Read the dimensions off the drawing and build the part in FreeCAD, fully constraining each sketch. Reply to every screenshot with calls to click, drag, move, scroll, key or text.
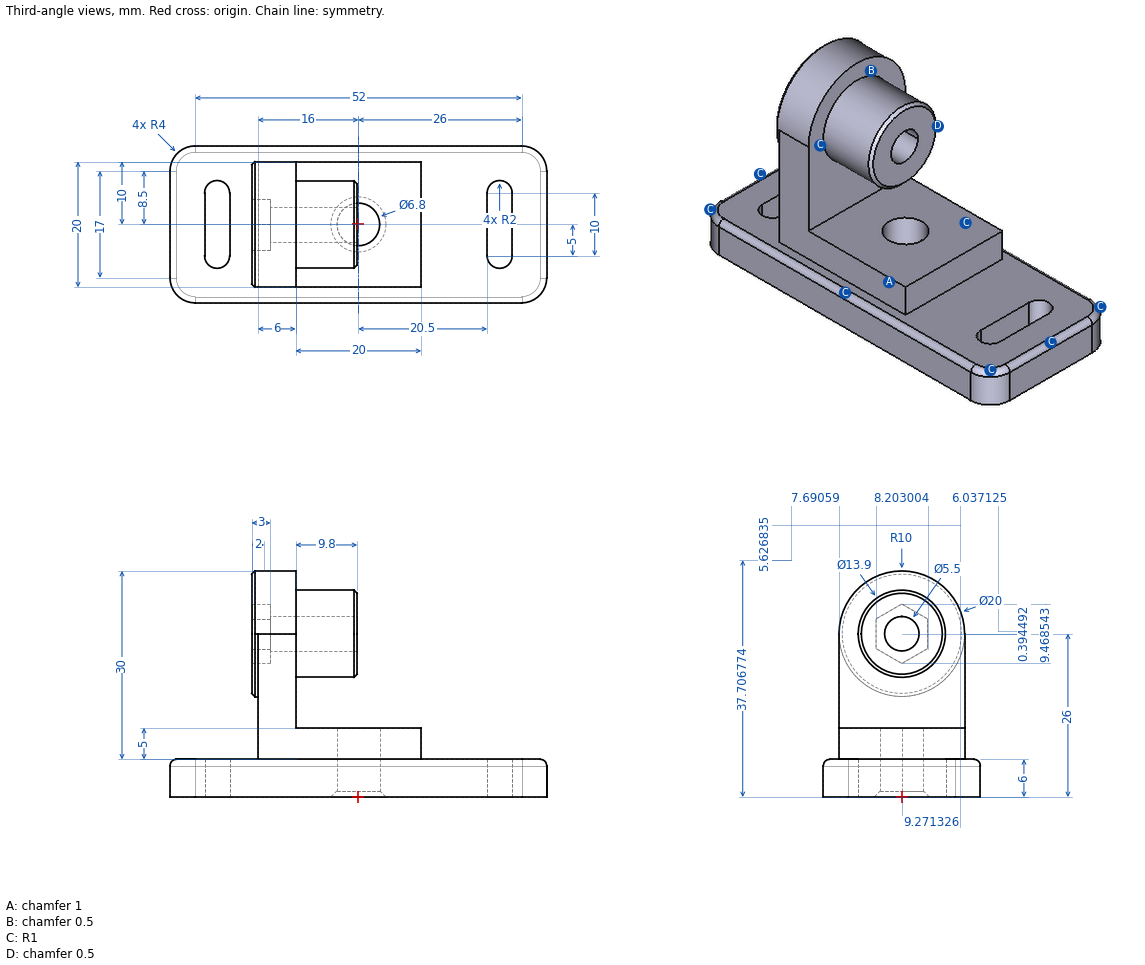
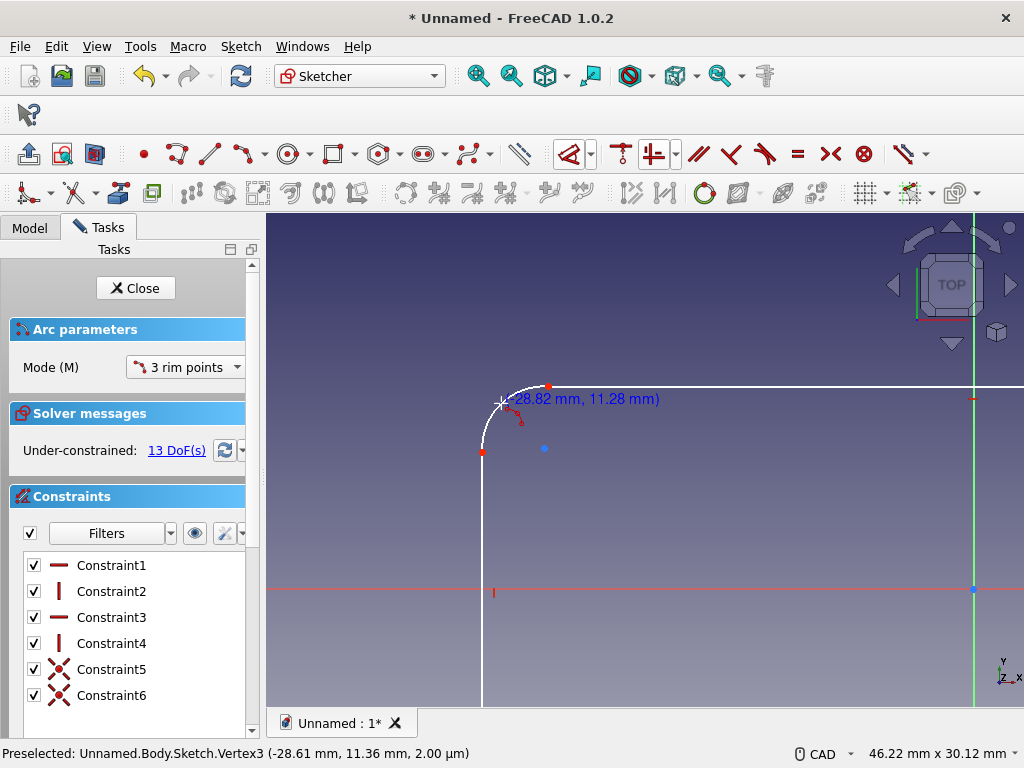
scroll(345, 385, down, 5)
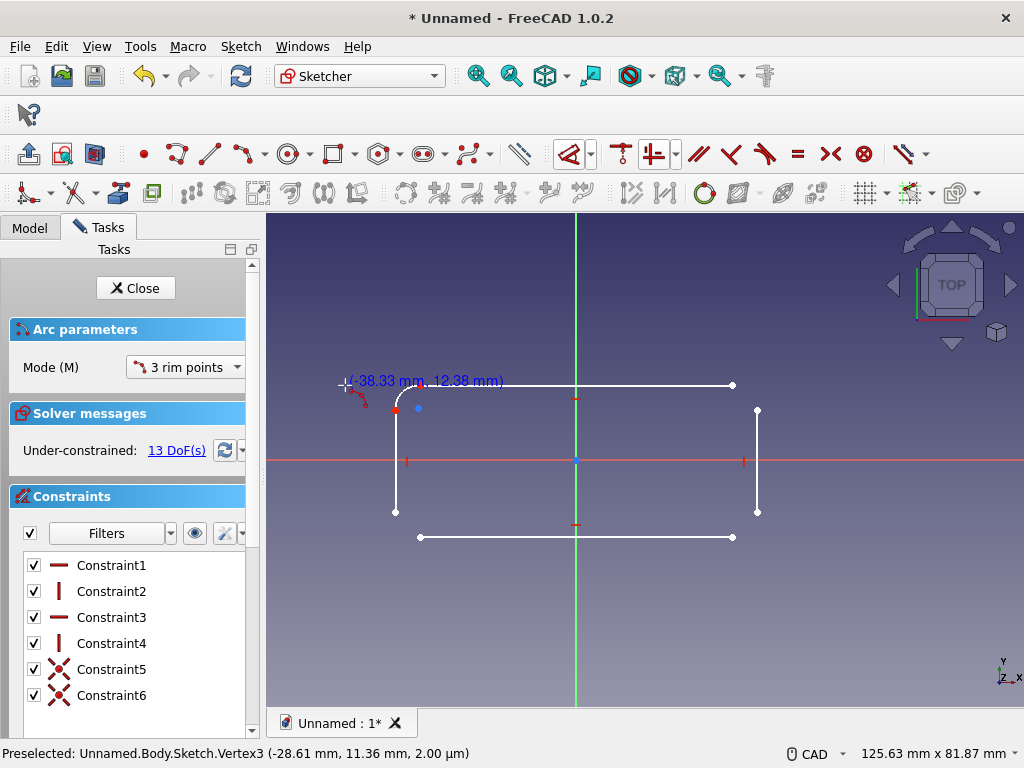
click(396, 513)
click(420, 537)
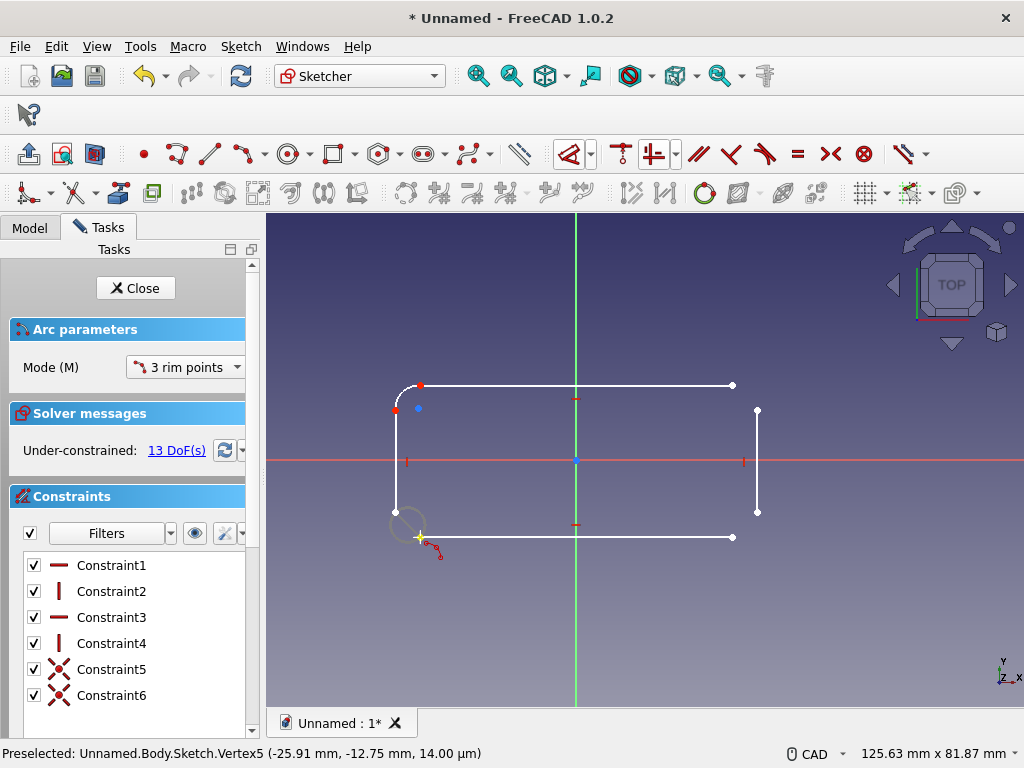
scroll(402, 529, up, 5)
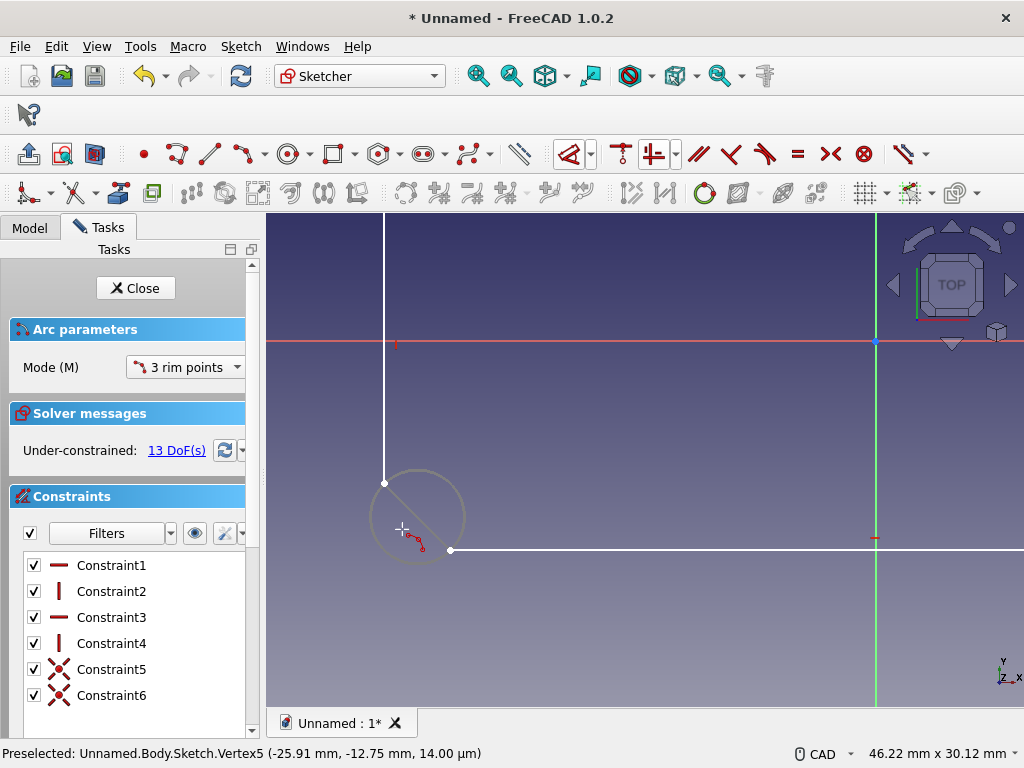
click(403, 527)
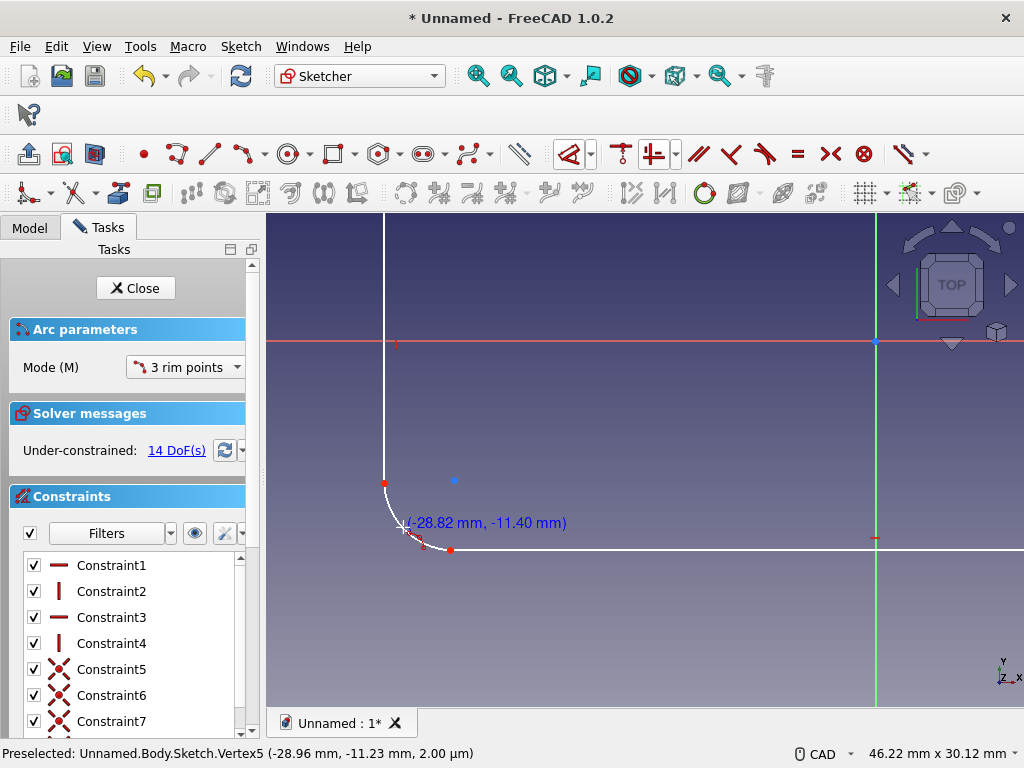
scroll(402, 529, down, 5)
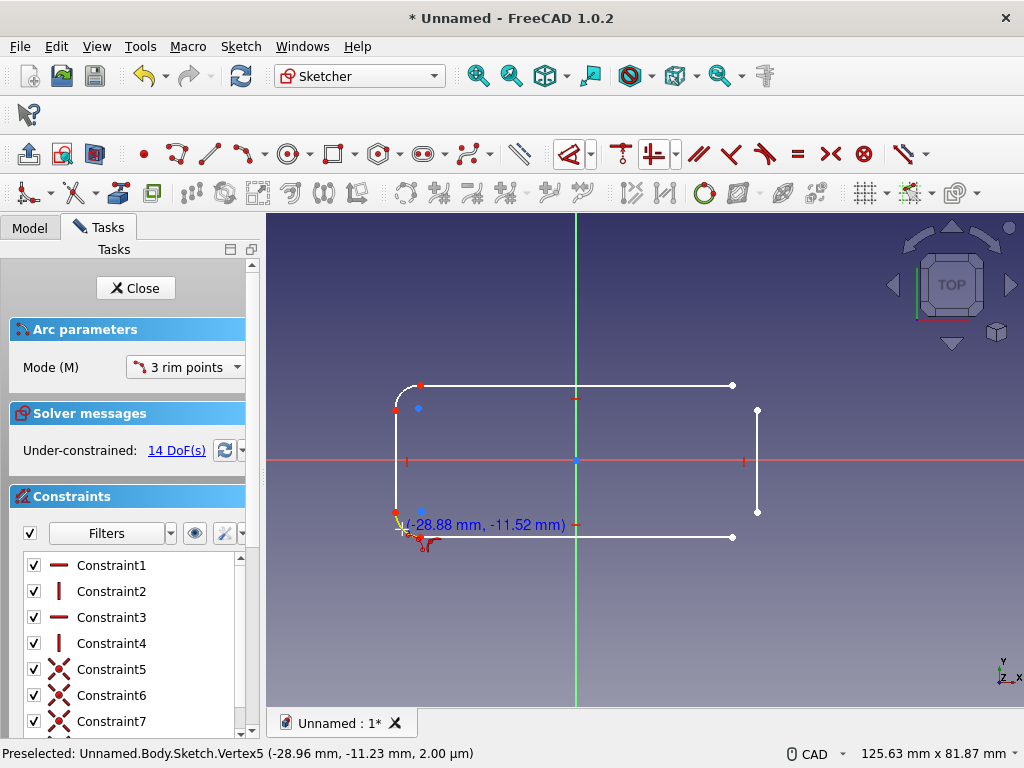
click(733, 537)
click(757, 513)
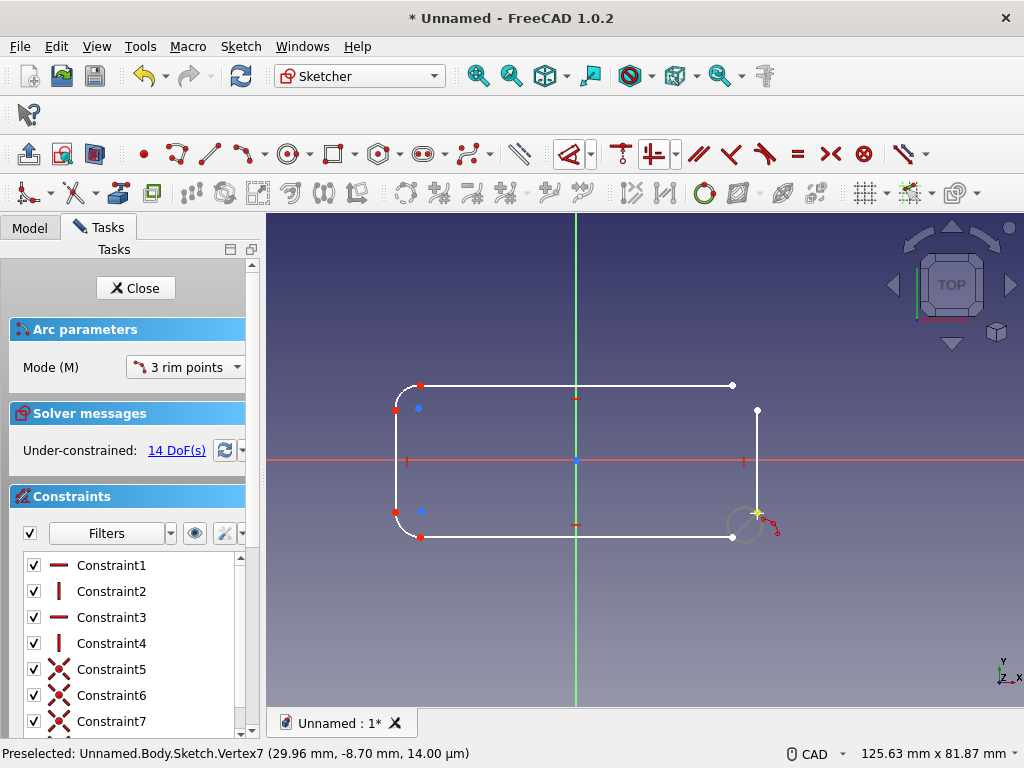
scroll(750, 529, up, 5)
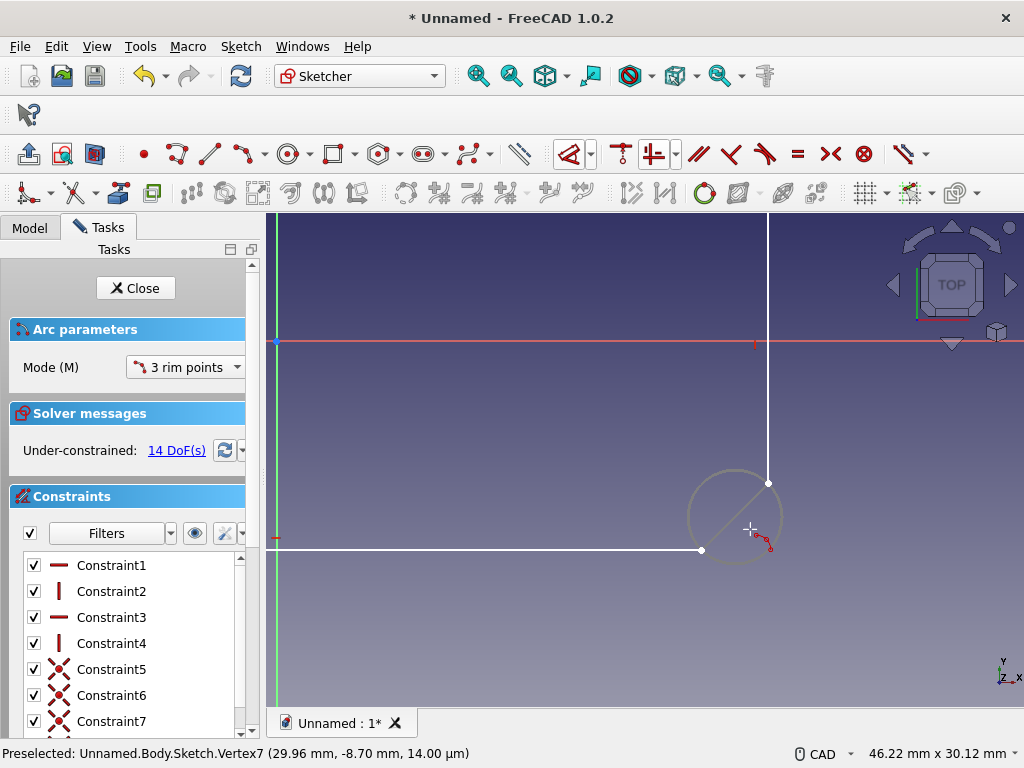
click(750, 527)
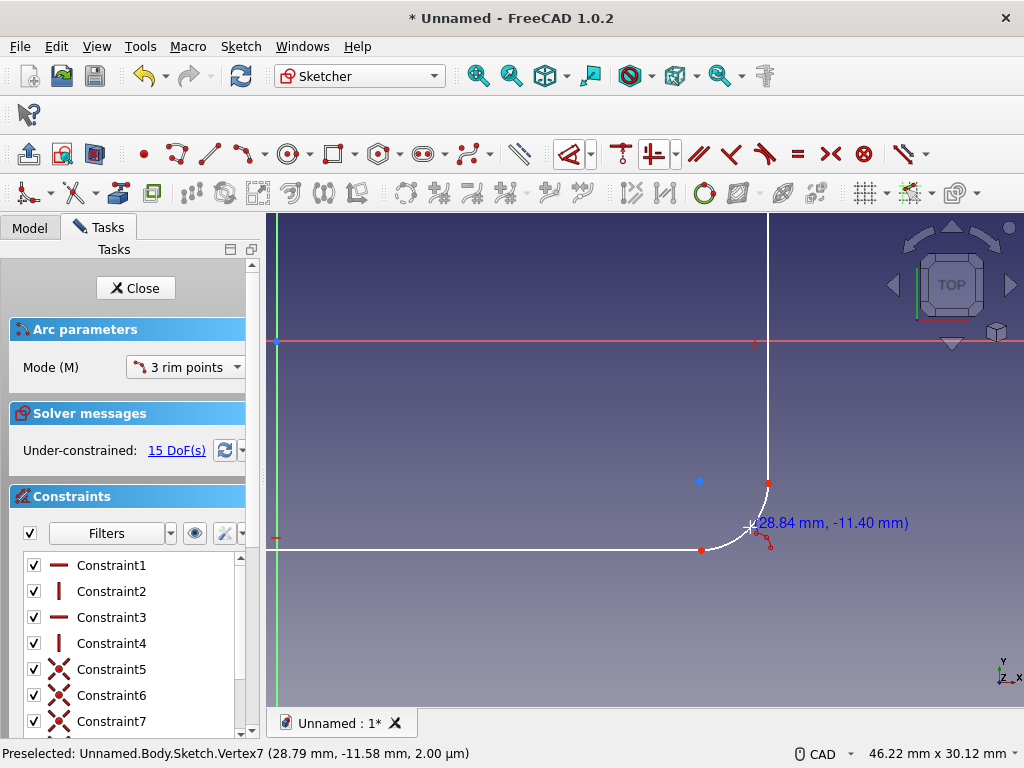
scroll(751, 529, down, 5)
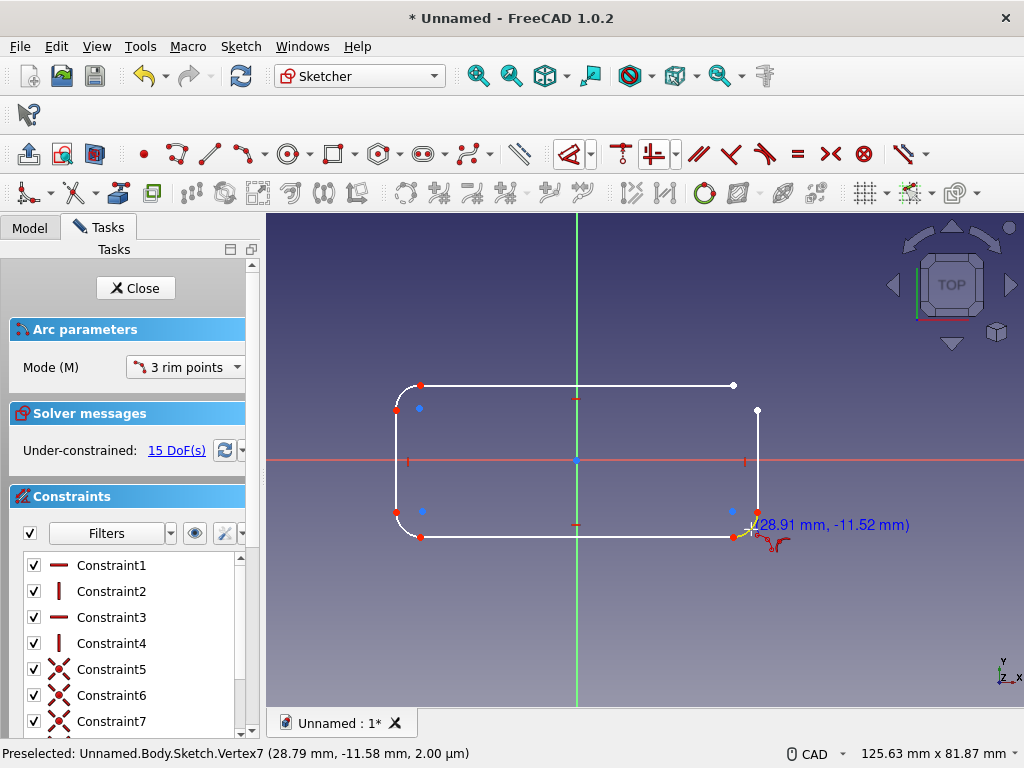
click(758, 410)
click(733, 386)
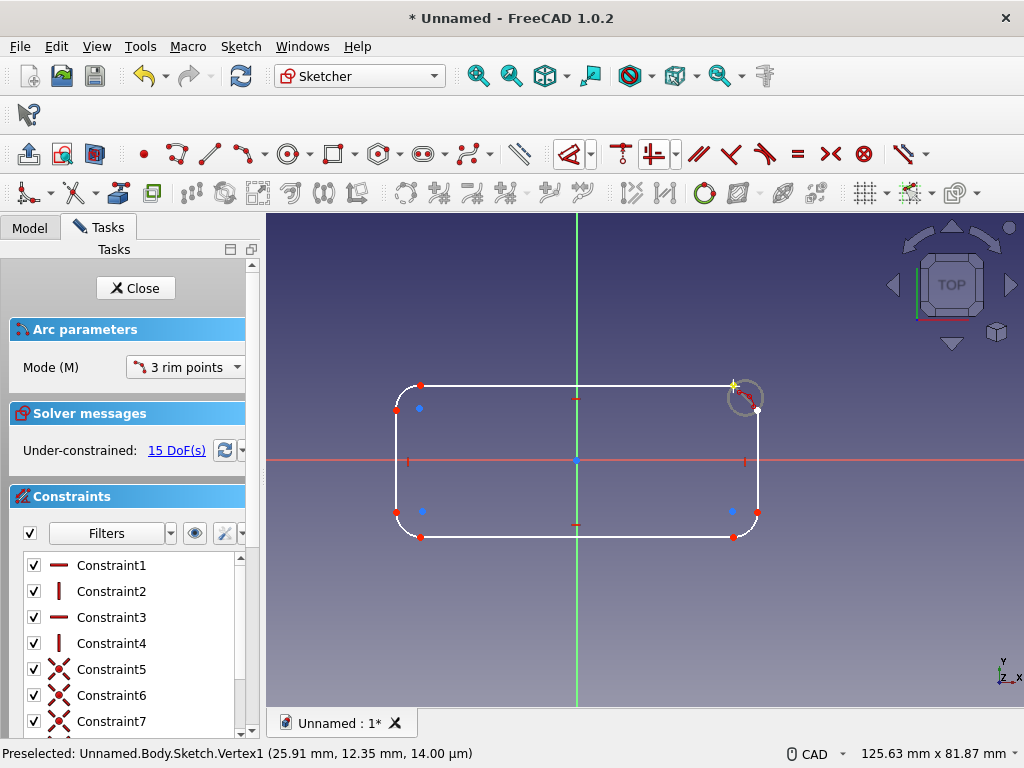
scroll(751, 392, up, 5)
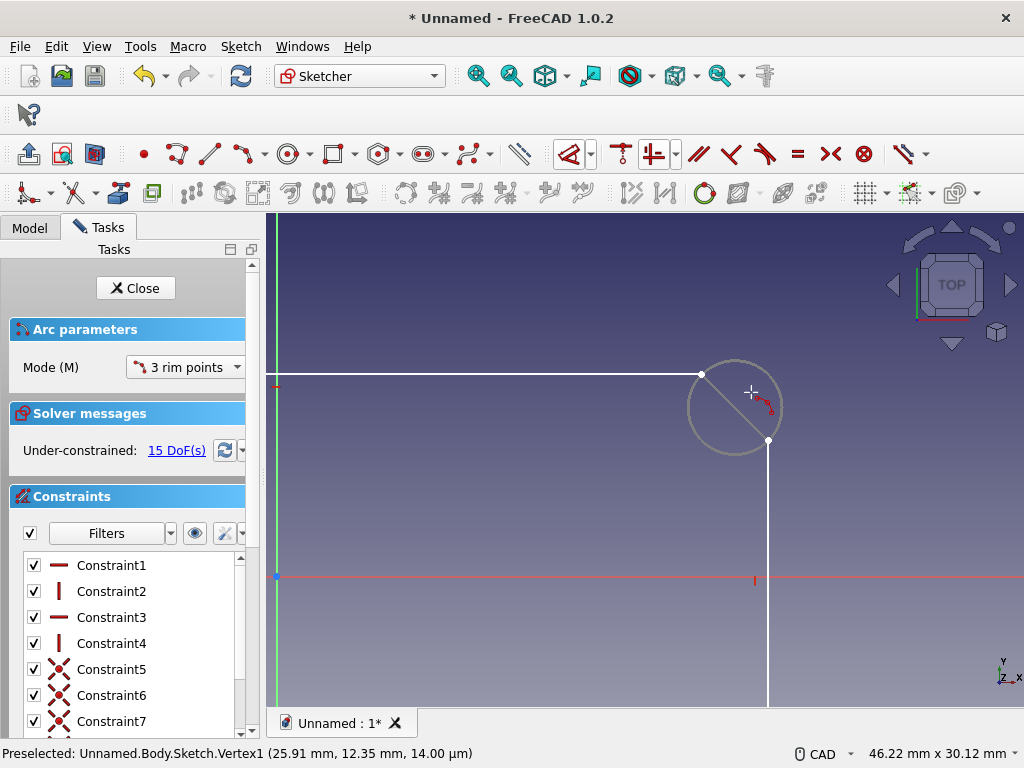
click(750, 391)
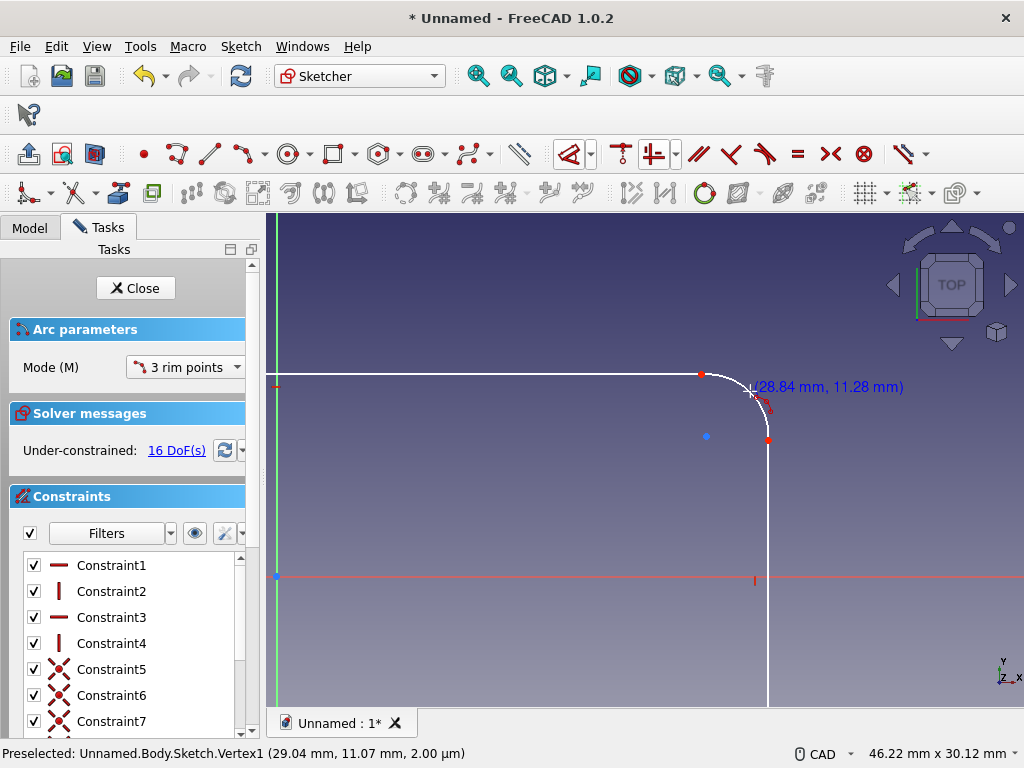
click(422, 154)